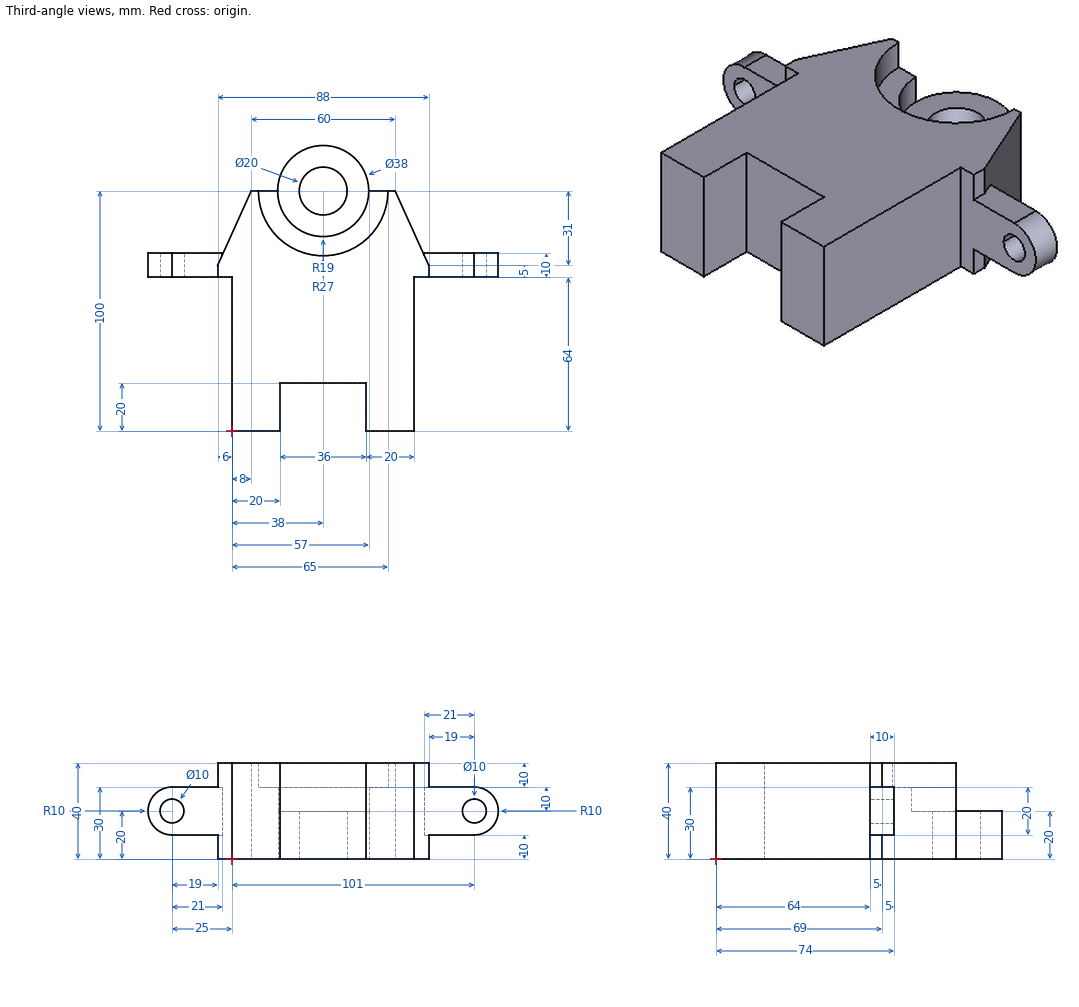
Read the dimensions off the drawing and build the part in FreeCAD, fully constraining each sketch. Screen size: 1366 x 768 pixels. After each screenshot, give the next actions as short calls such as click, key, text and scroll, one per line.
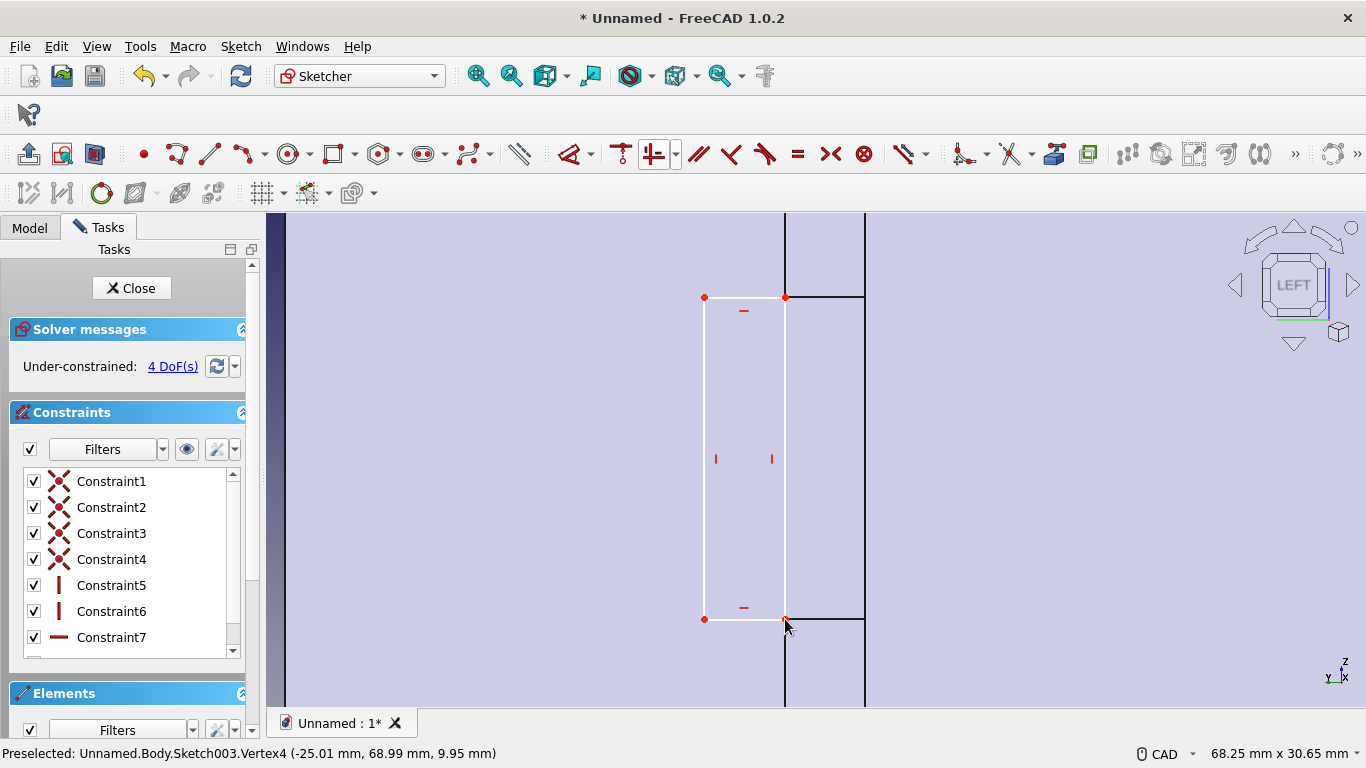
click(568, 154)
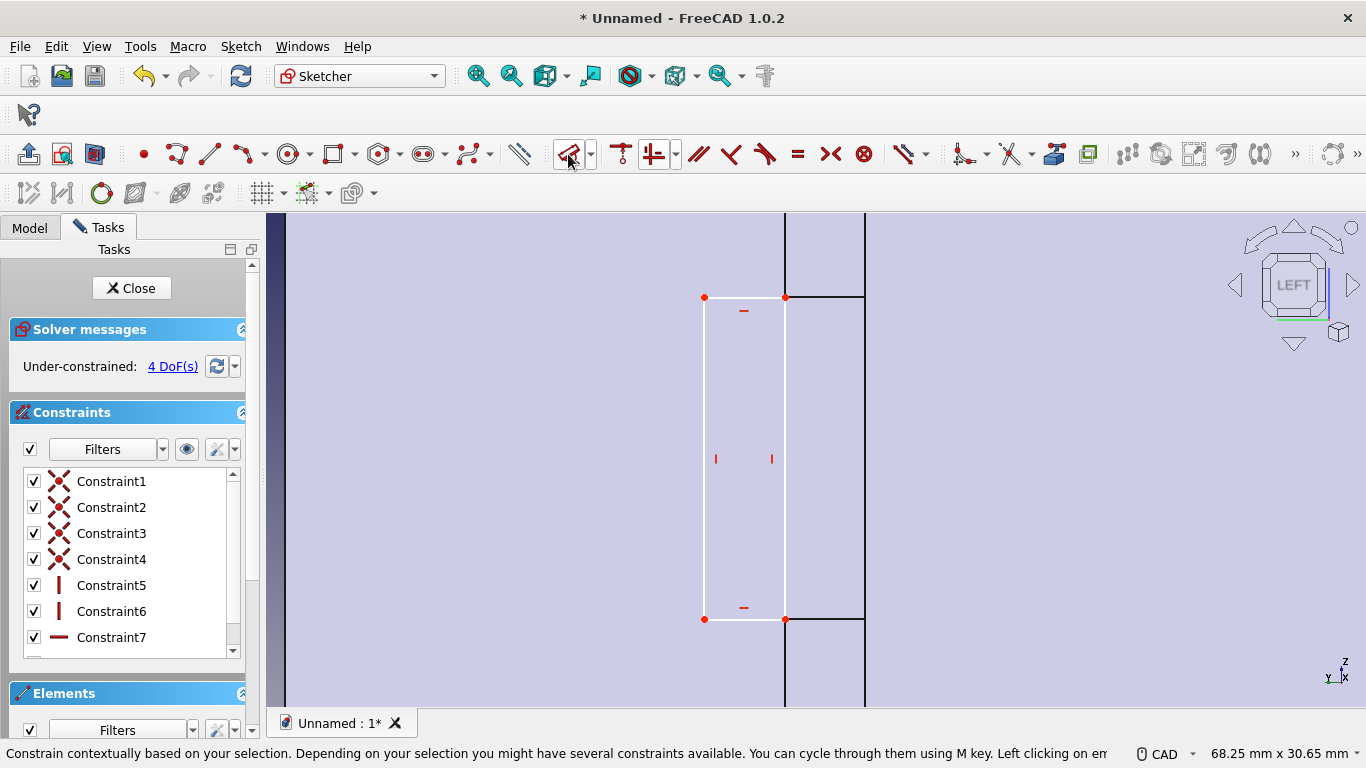
click(728, 620)
click(744, 654)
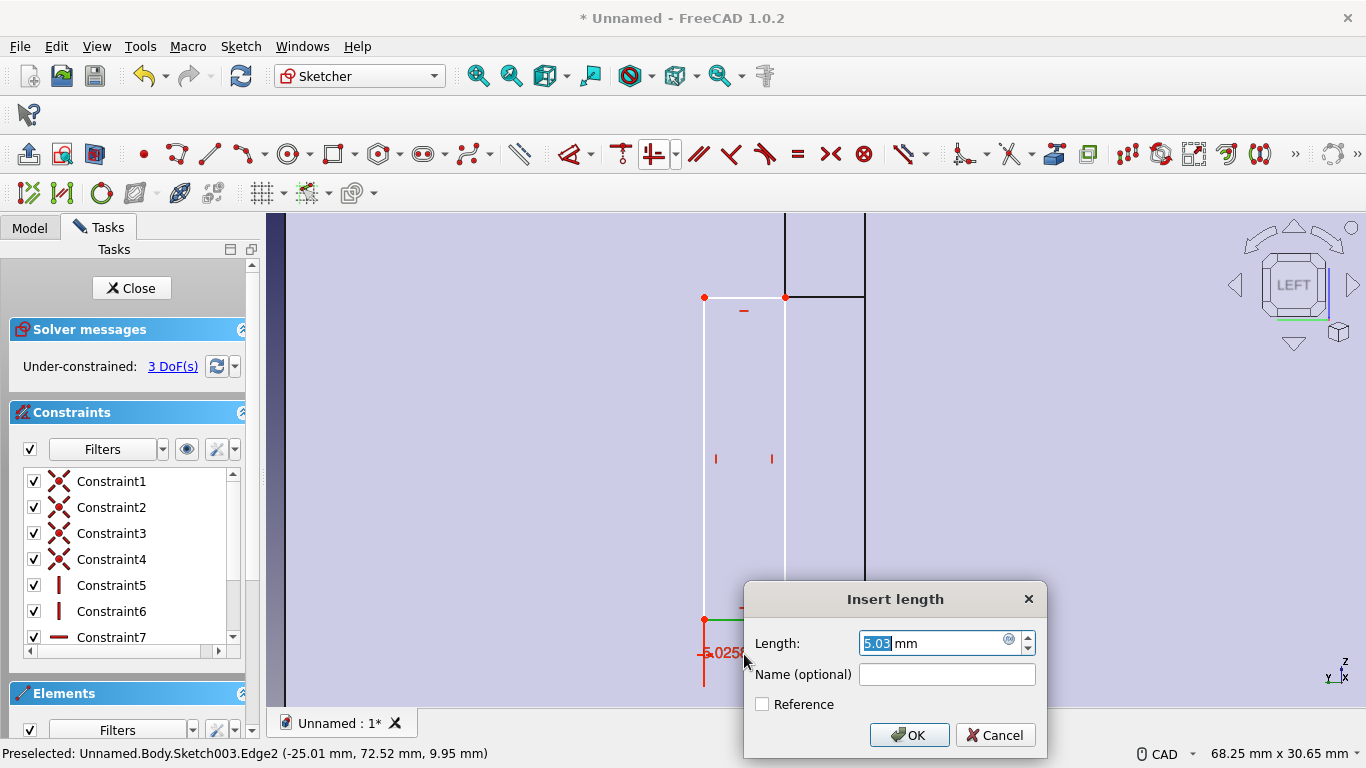
text(5)
key(Return)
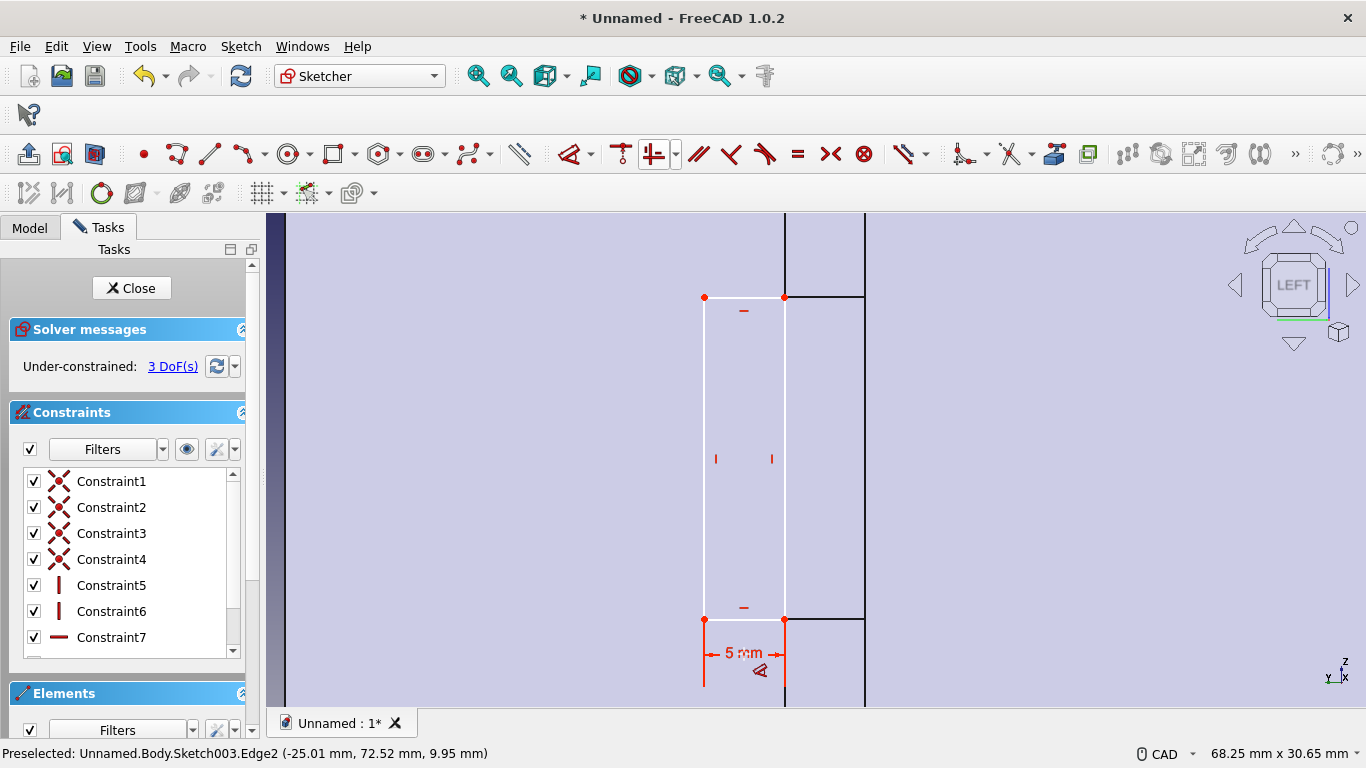
click(704, 395)
click(670, 459)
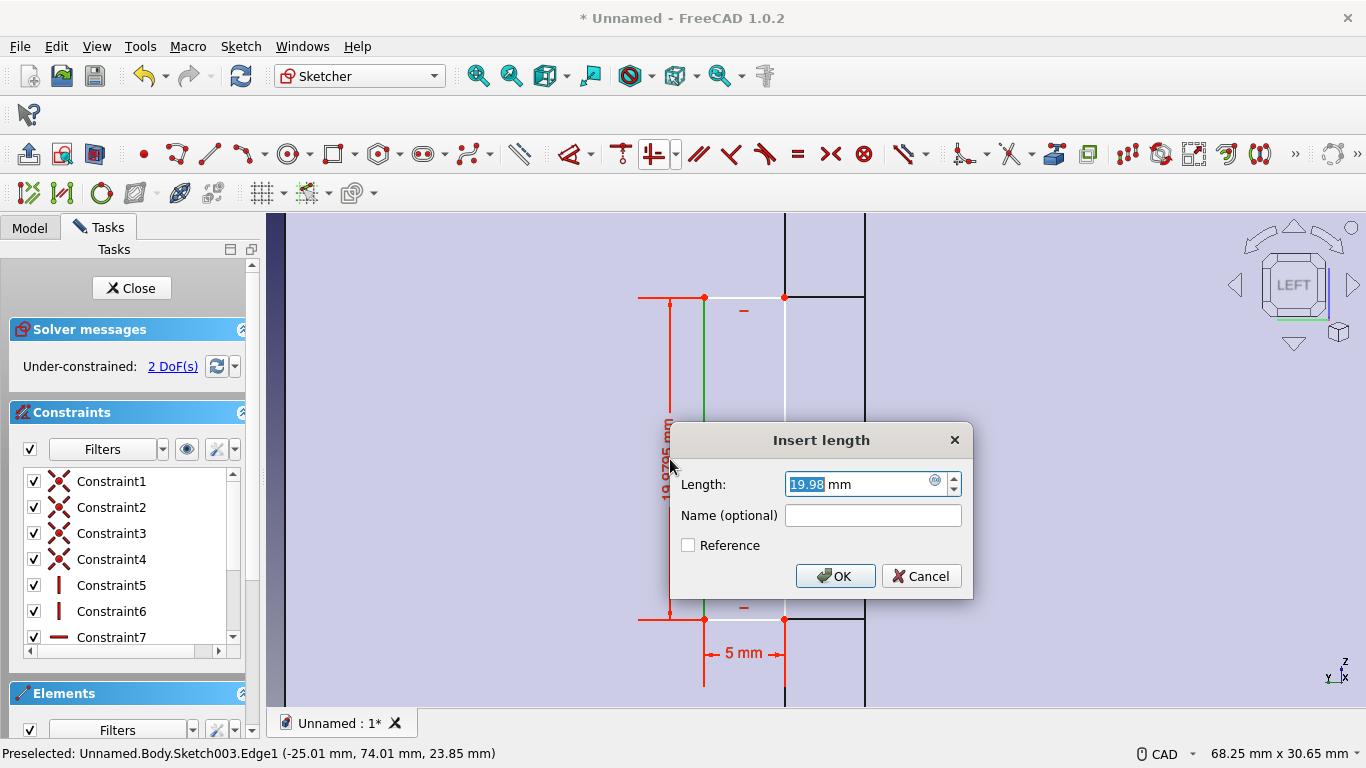
text(20)
key(Return)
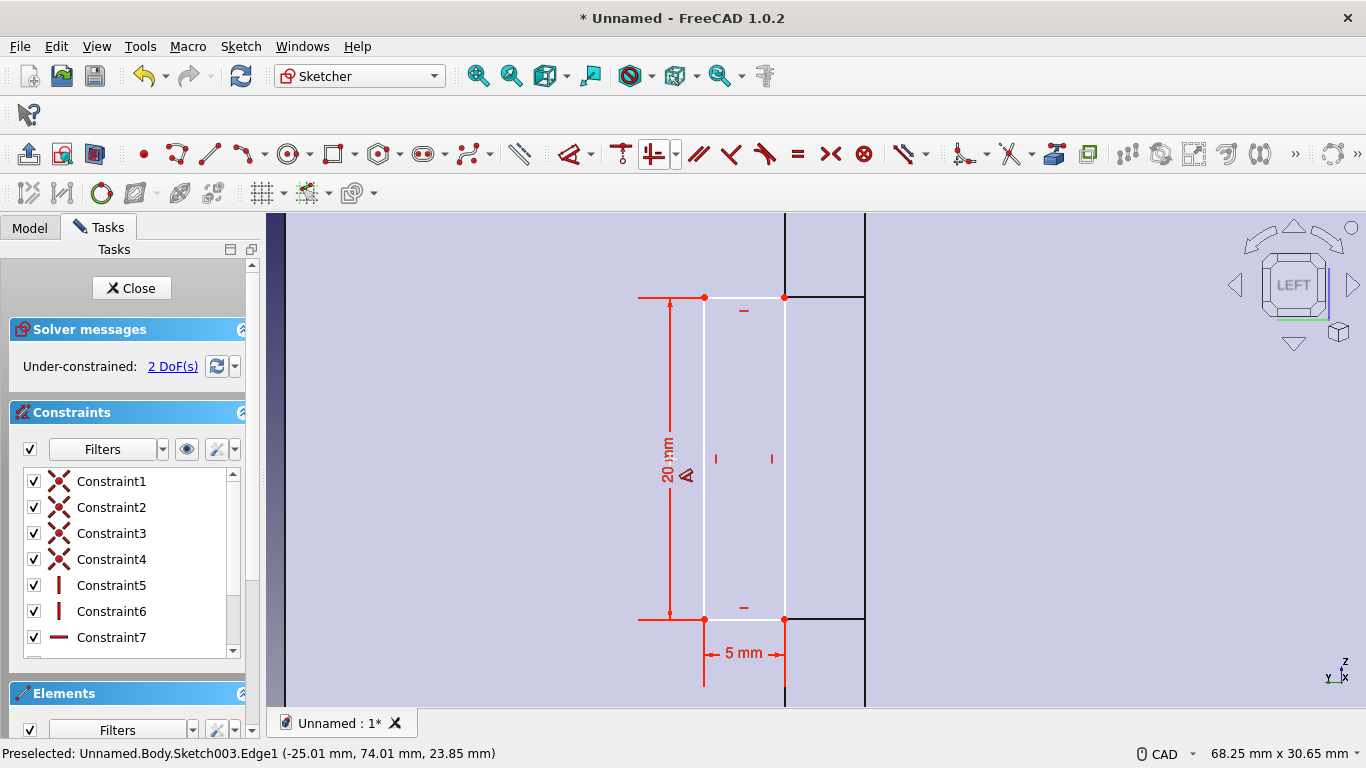
click(704, 298)
click(953, 264)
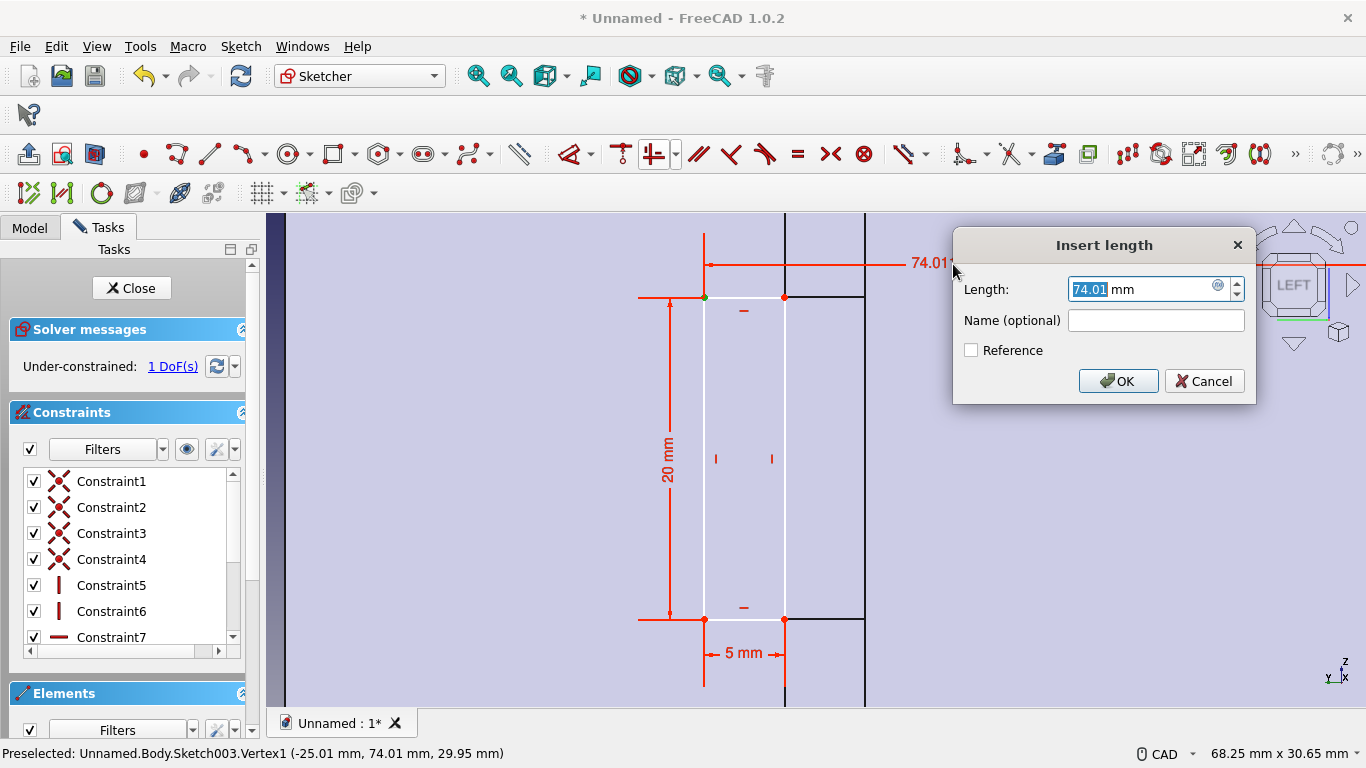
text(74)
key(Return)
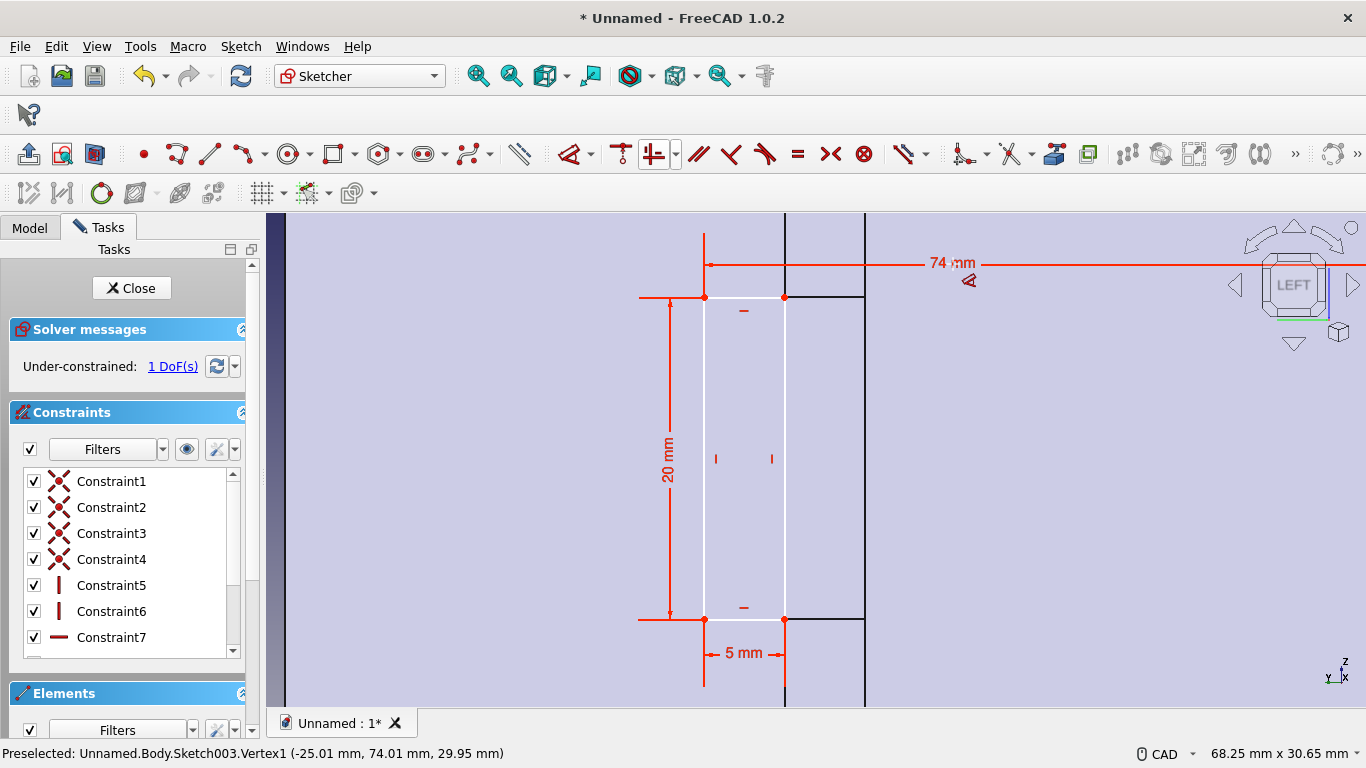
click(704, 298)
click(670, 488)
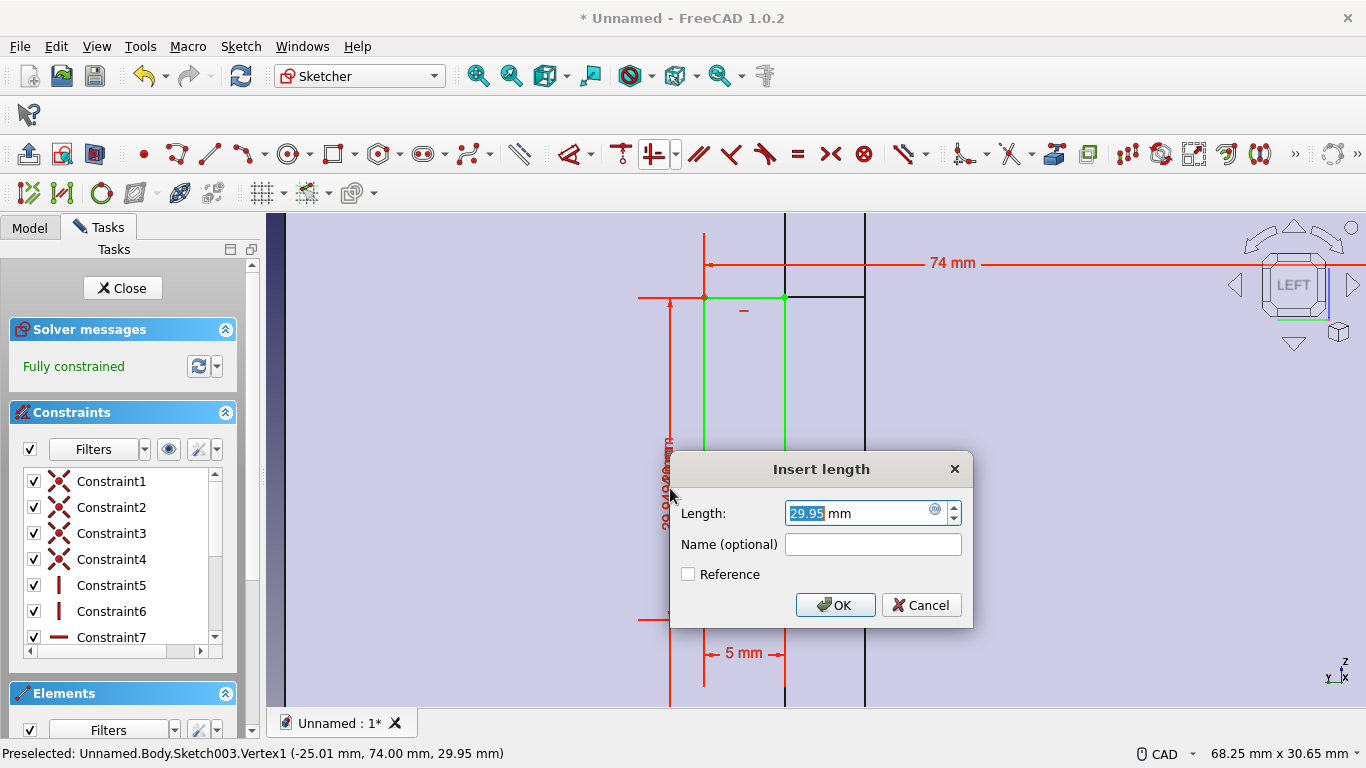
text(30)
key(Return)
key(Escape)